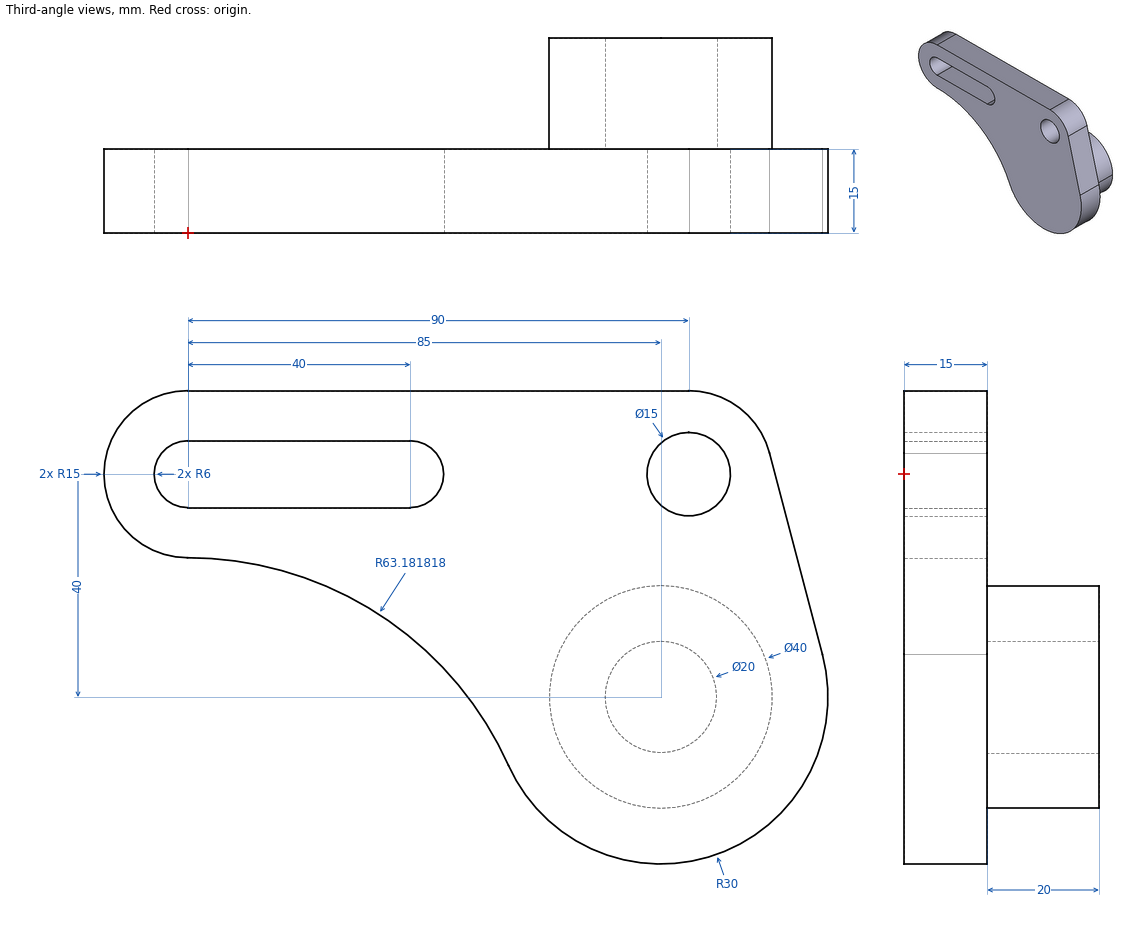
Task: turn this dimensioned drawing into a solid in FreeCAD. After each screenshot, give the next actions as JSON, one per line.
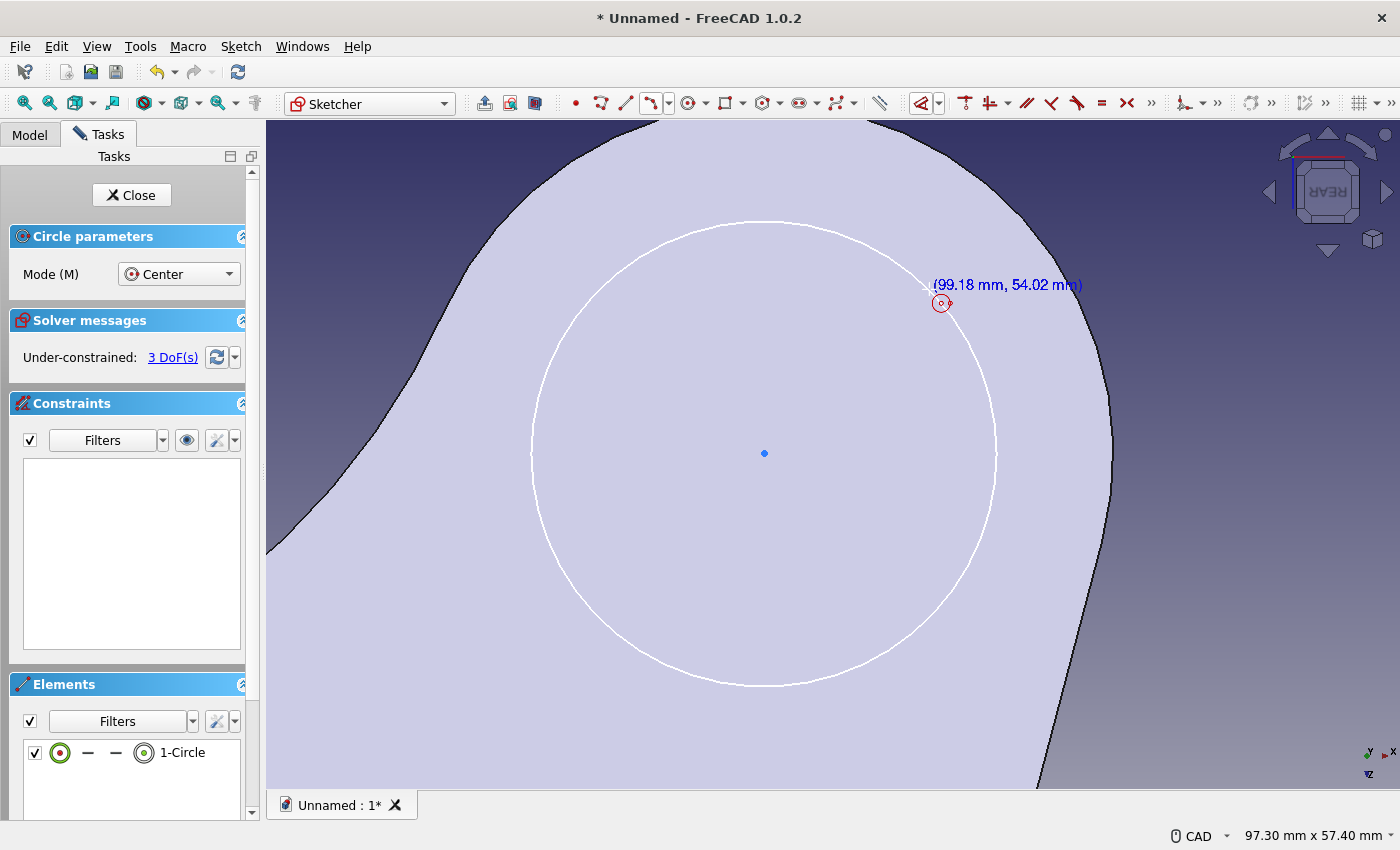
{"action": "left_click", "coordinate": [764, 454]}
{"action": "left_click", "coordinate": [846, 371]}
{"action": "key", "text": "Escape"}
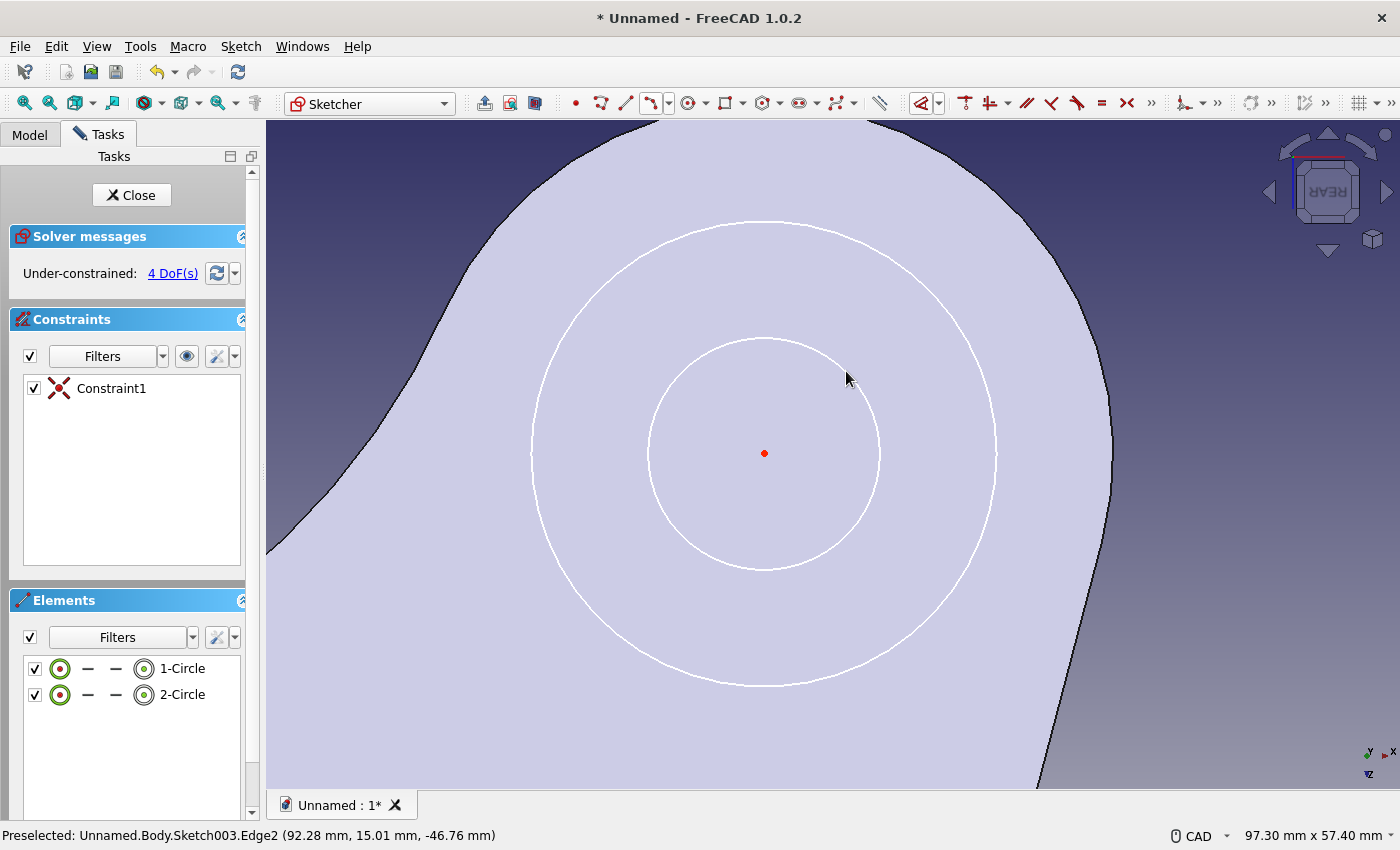
{"action": "left_click", "coordinate": [928, 289]}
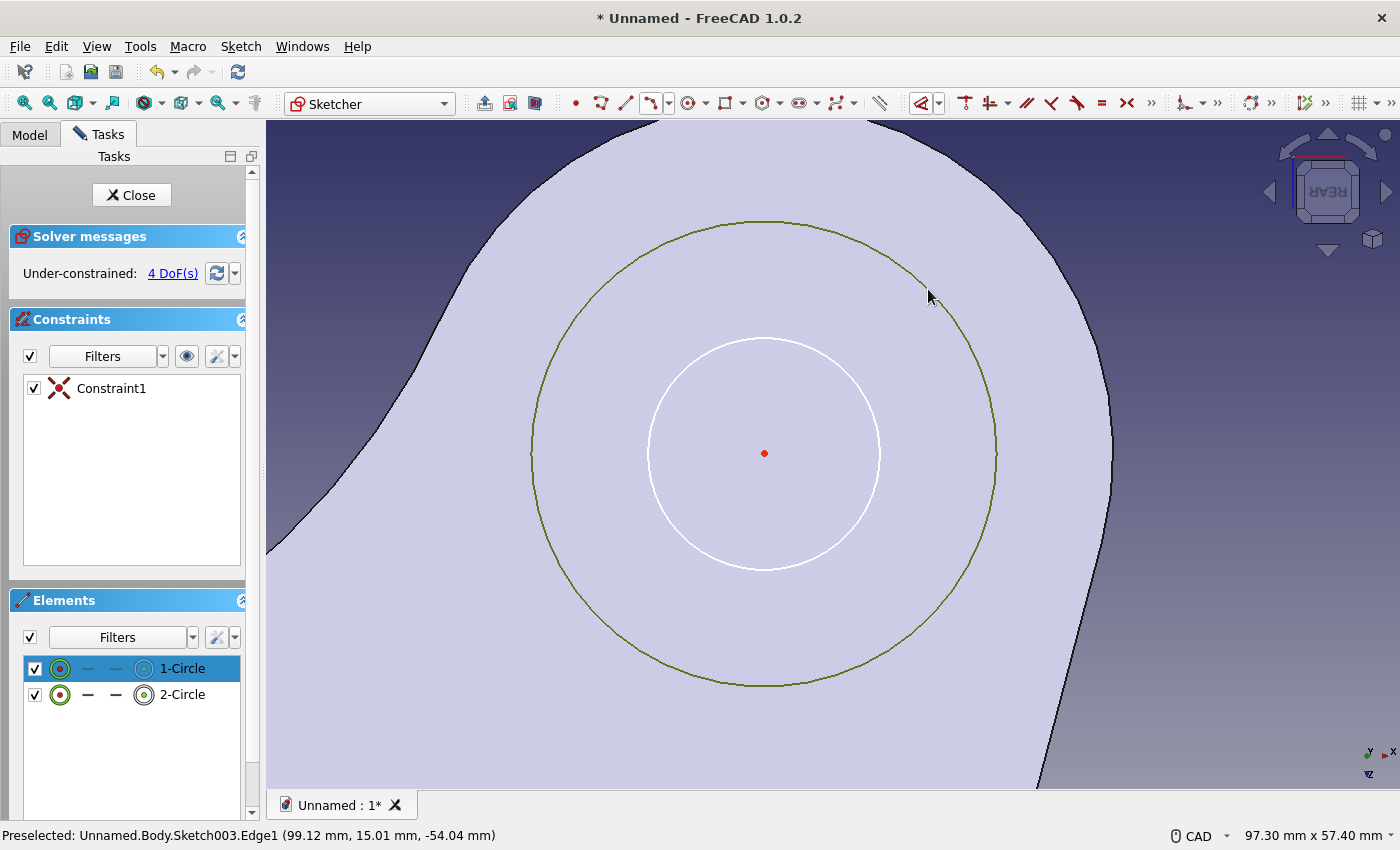
{"action": "left_click", "coordinate": [938, 104]}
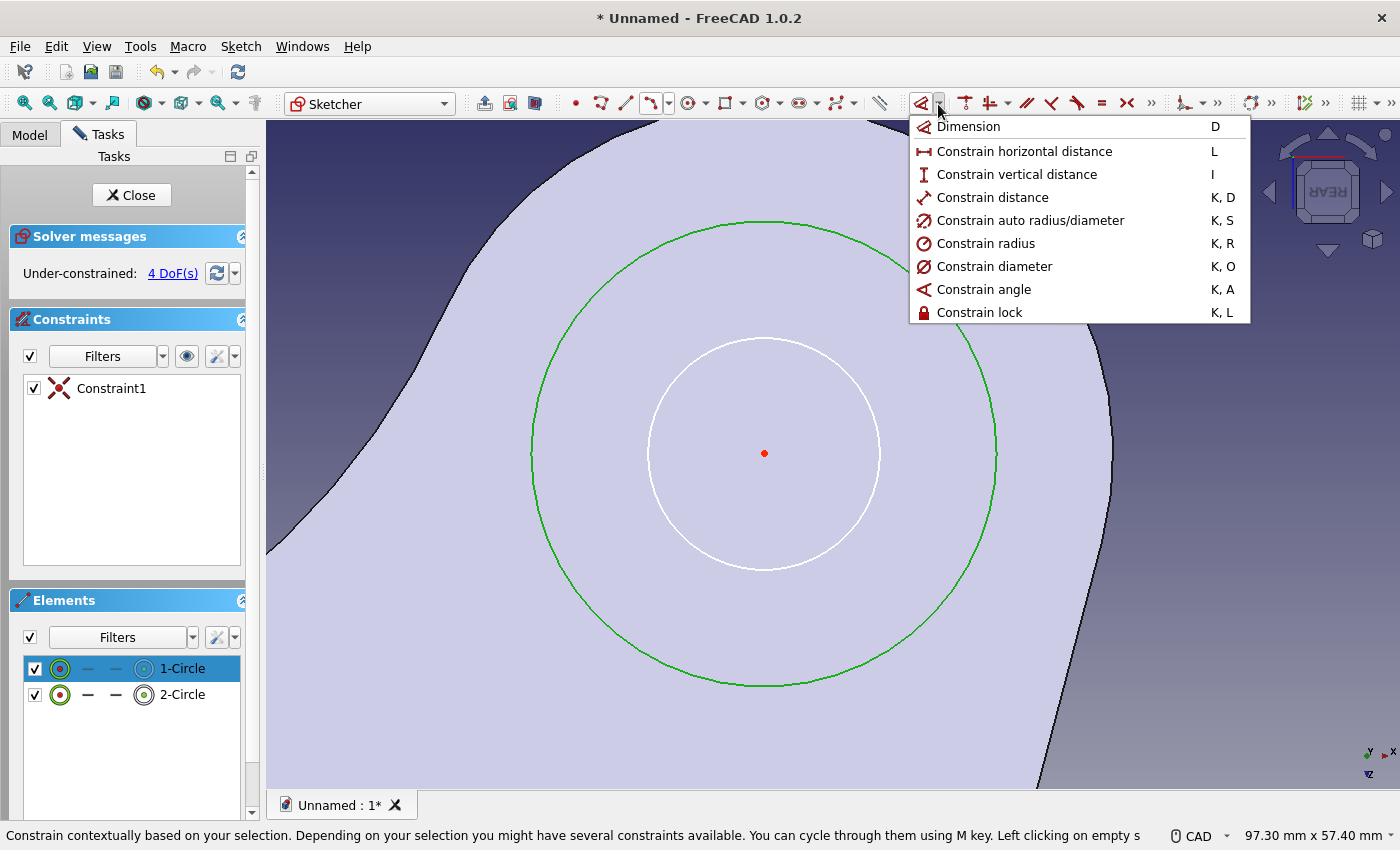
{"action": "left_click", "coordinate": [1080, 266]}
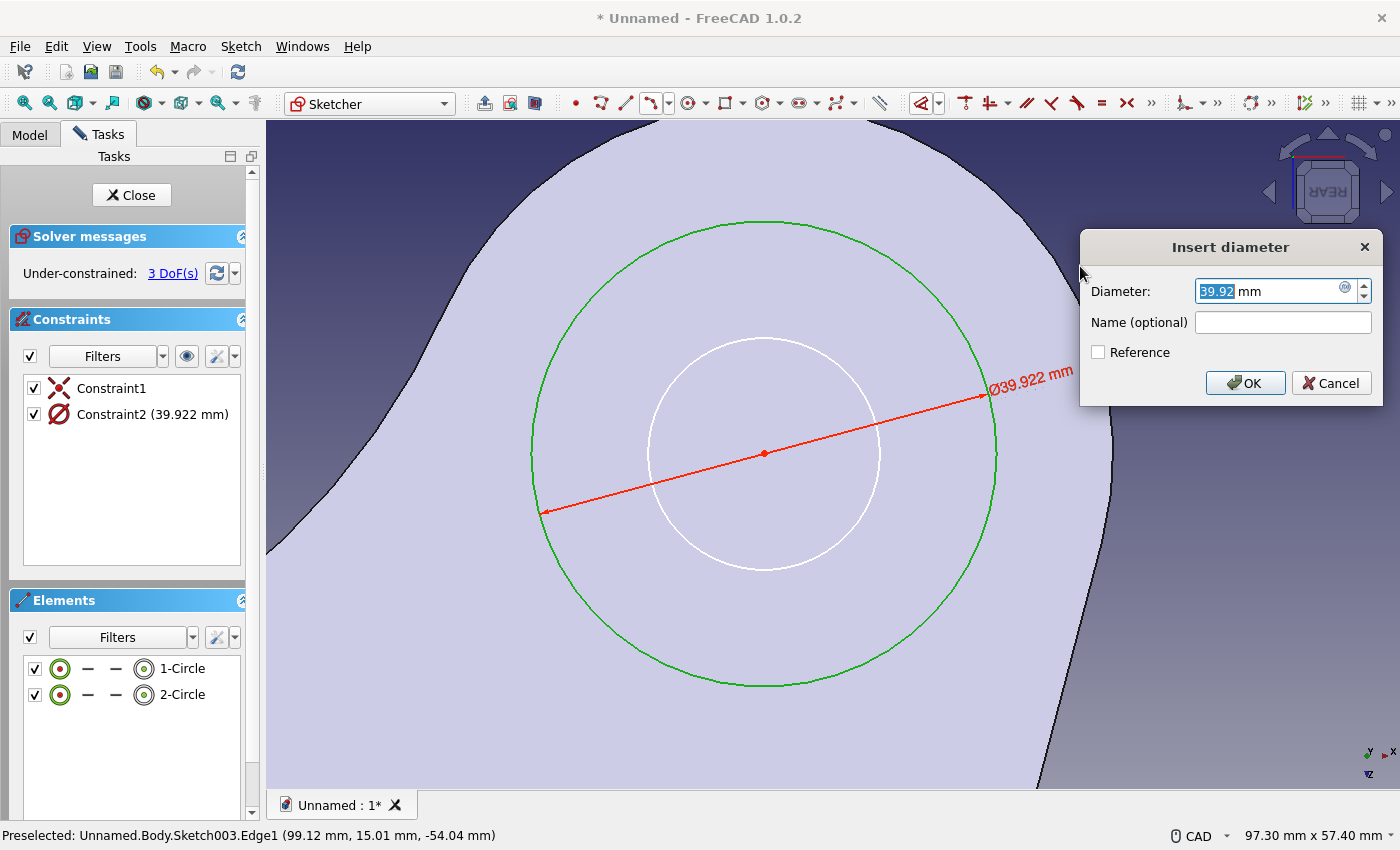
{"action": "type", "text": "40"}
{"action": "key", "text": "Return"}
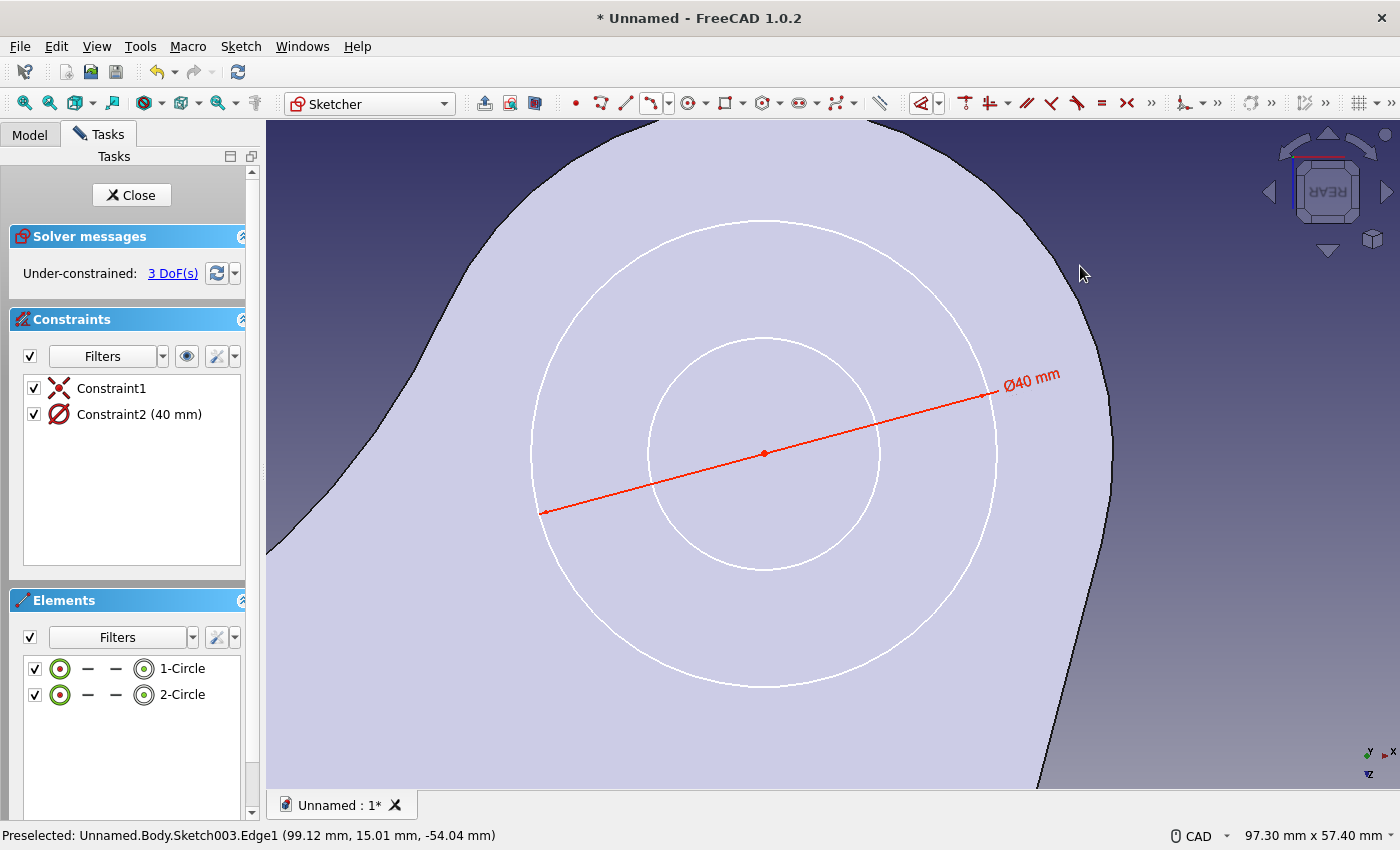
{"action": "left_click", "coordinate": [846, 372]}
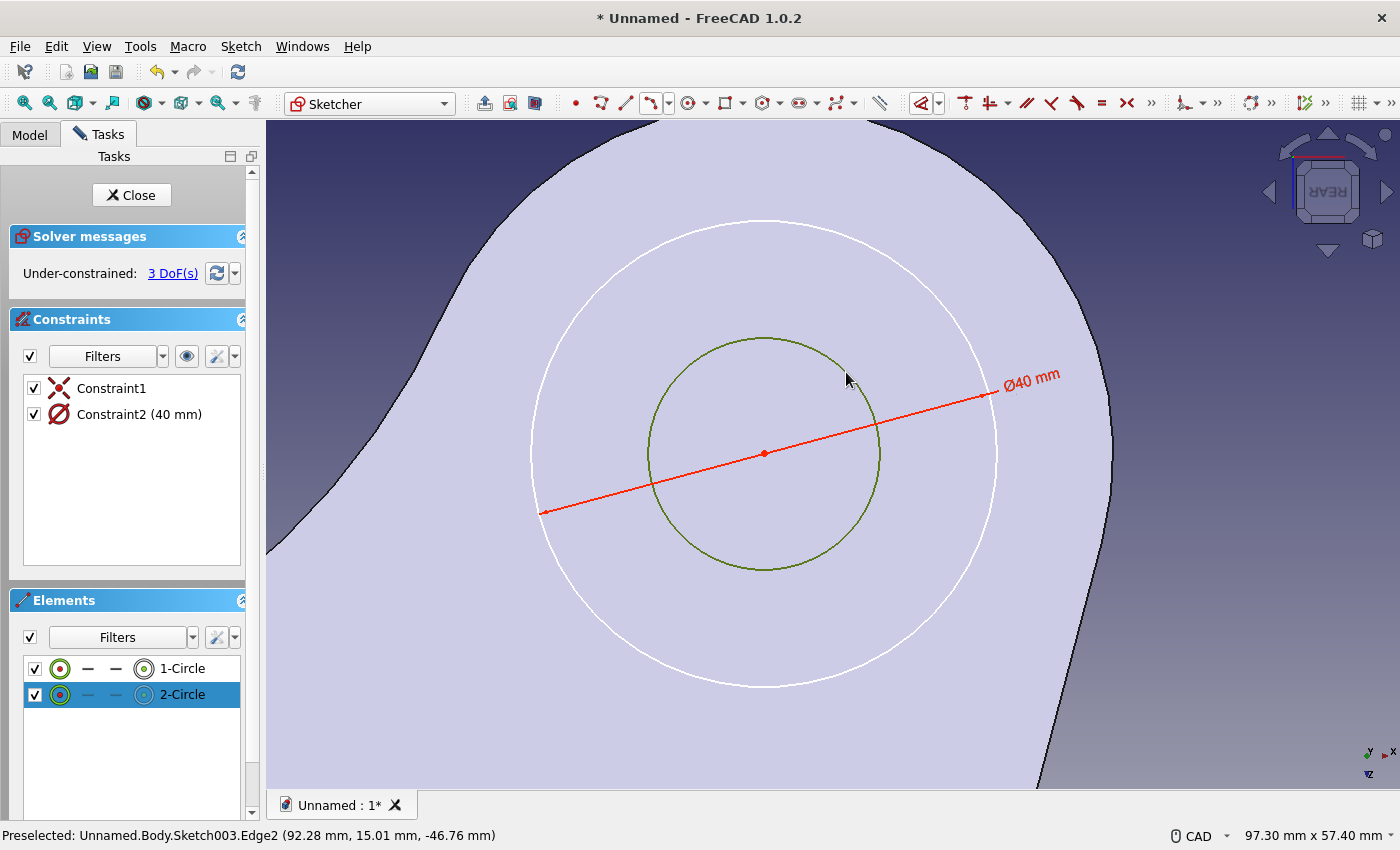
{"action": "left_click", "coordinate": [938, 104]}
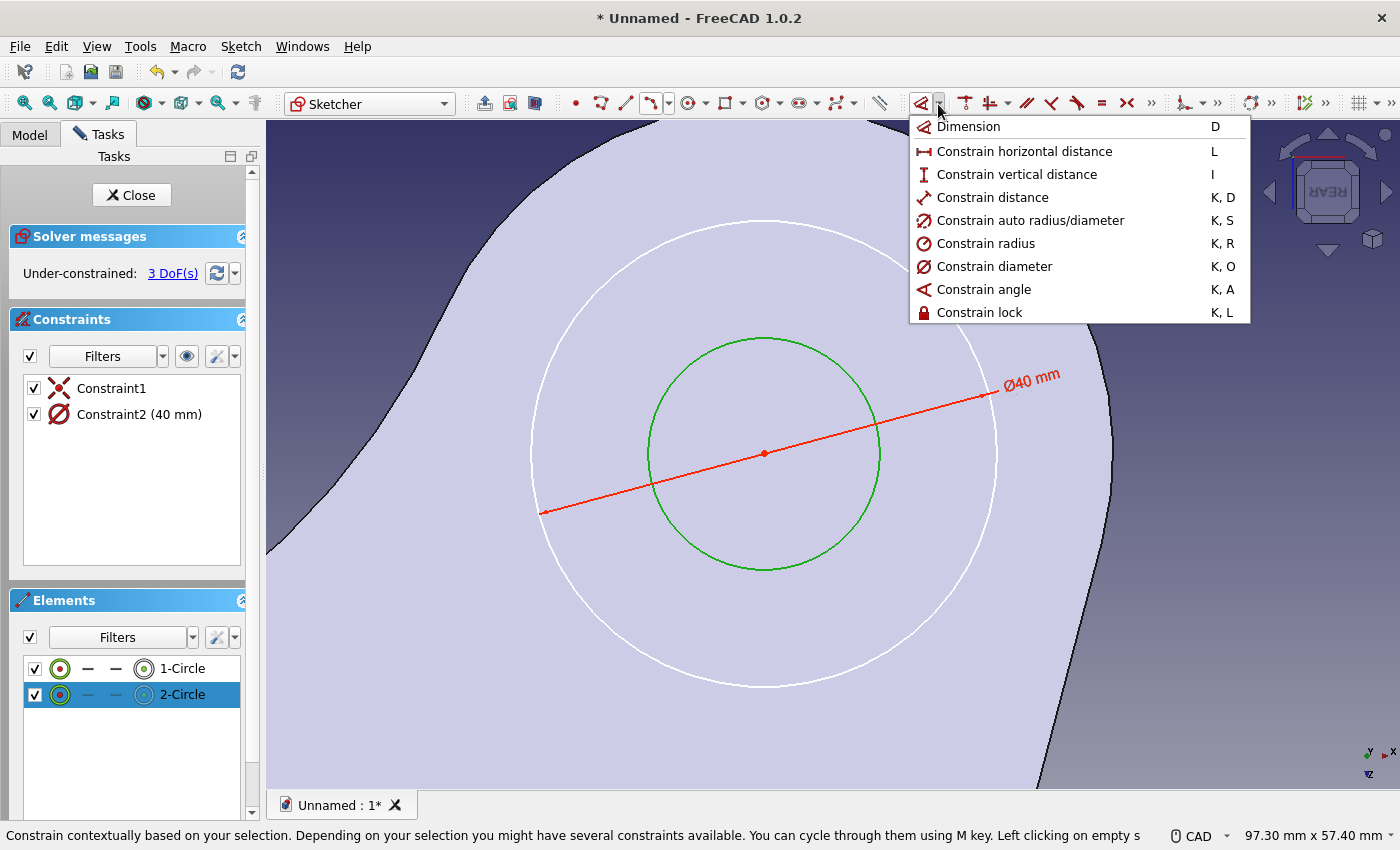
{"action": "left_click", "coordinate": [1080, 266]}